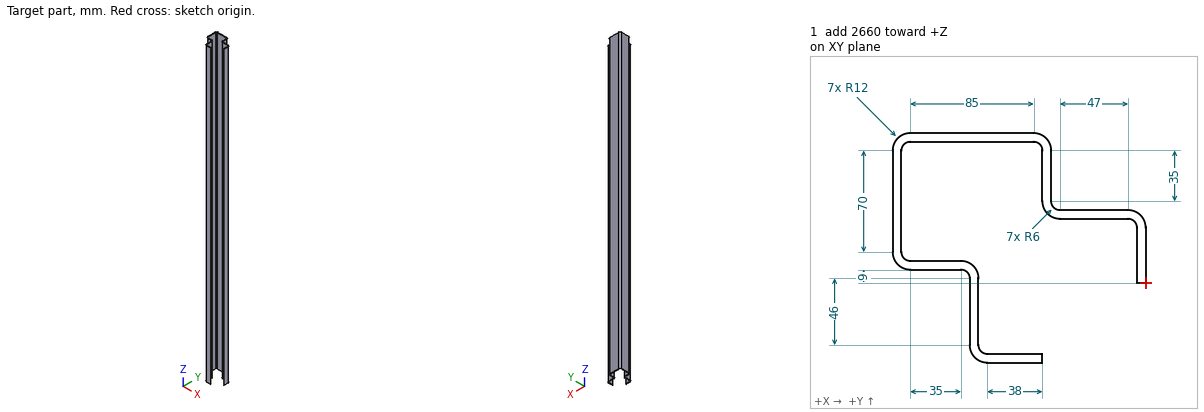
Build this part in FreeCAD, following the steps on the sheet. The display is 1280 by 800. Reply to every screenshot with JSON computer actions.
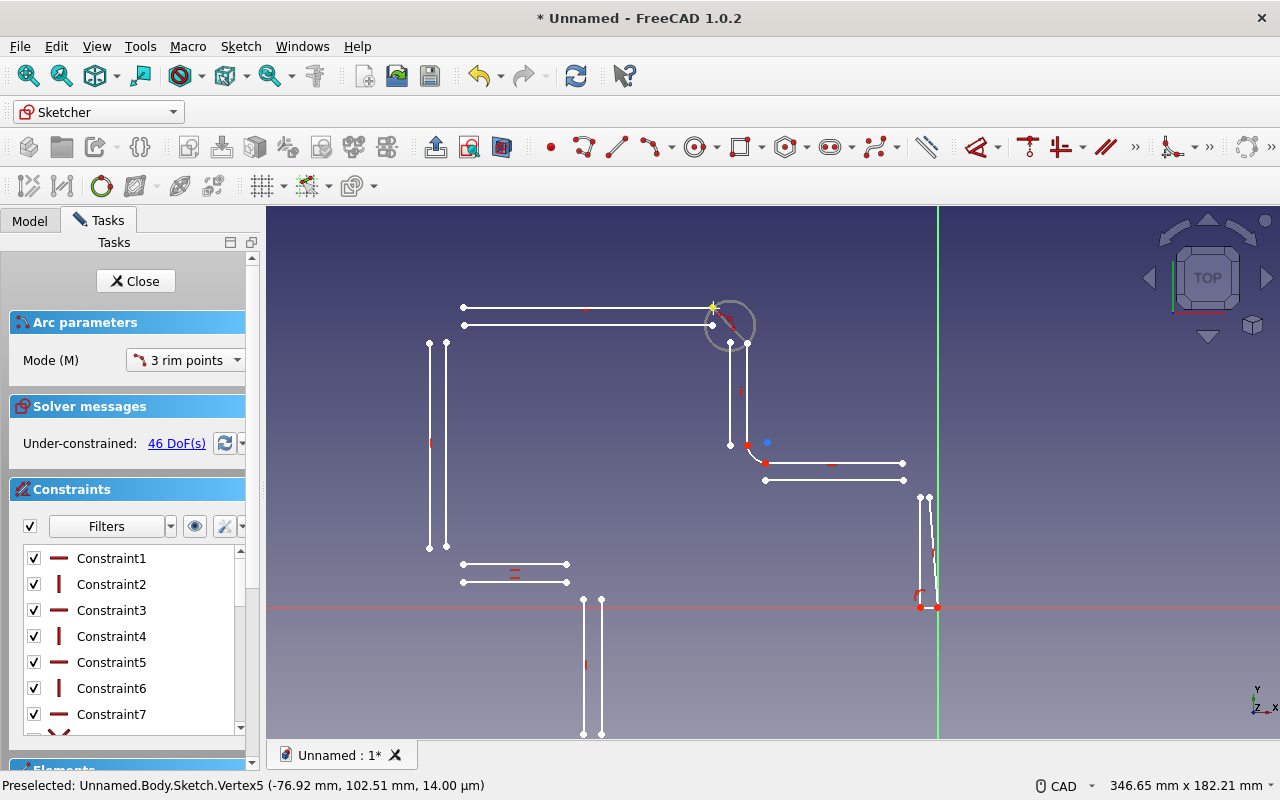
{"action": "scroll", "coordinate": [738, 317], "scroll_direction": "up", "scroll_amount": 3}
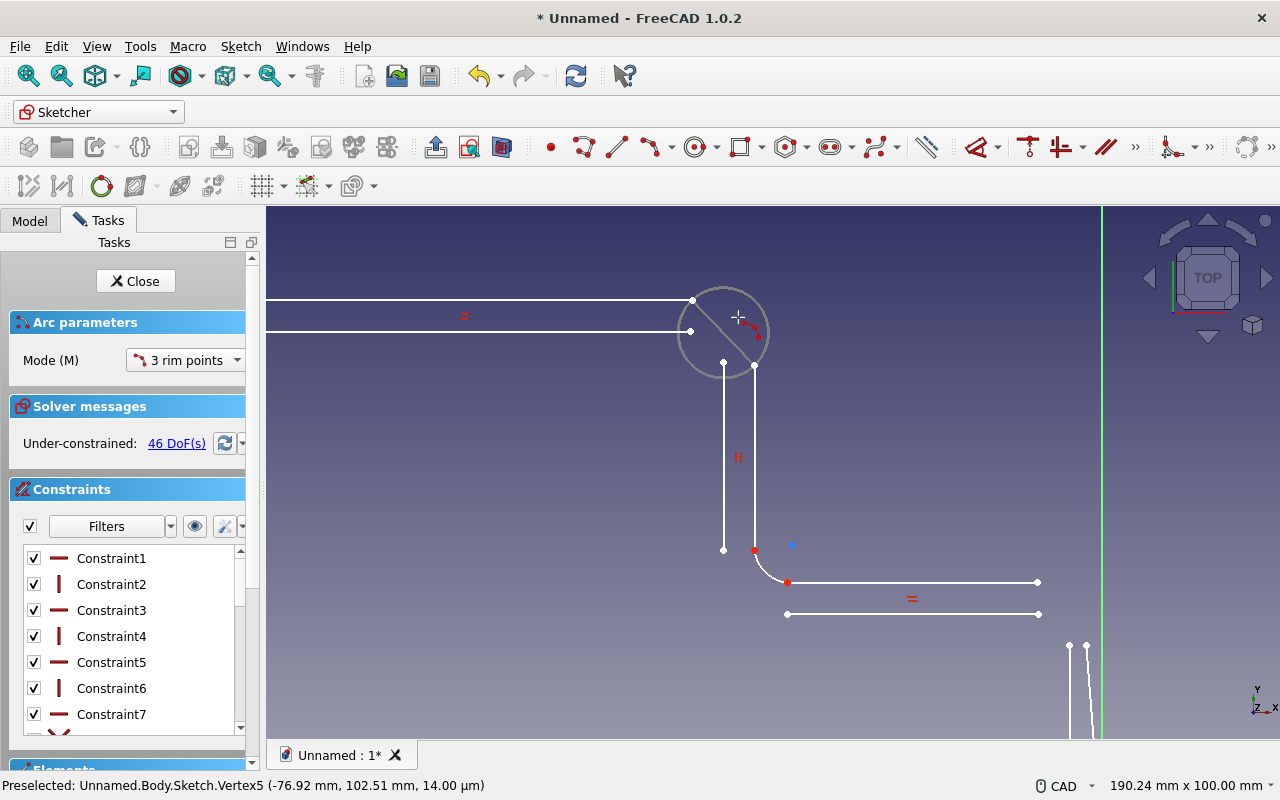
{"action": "left_click", "coordinate": [737, 316]}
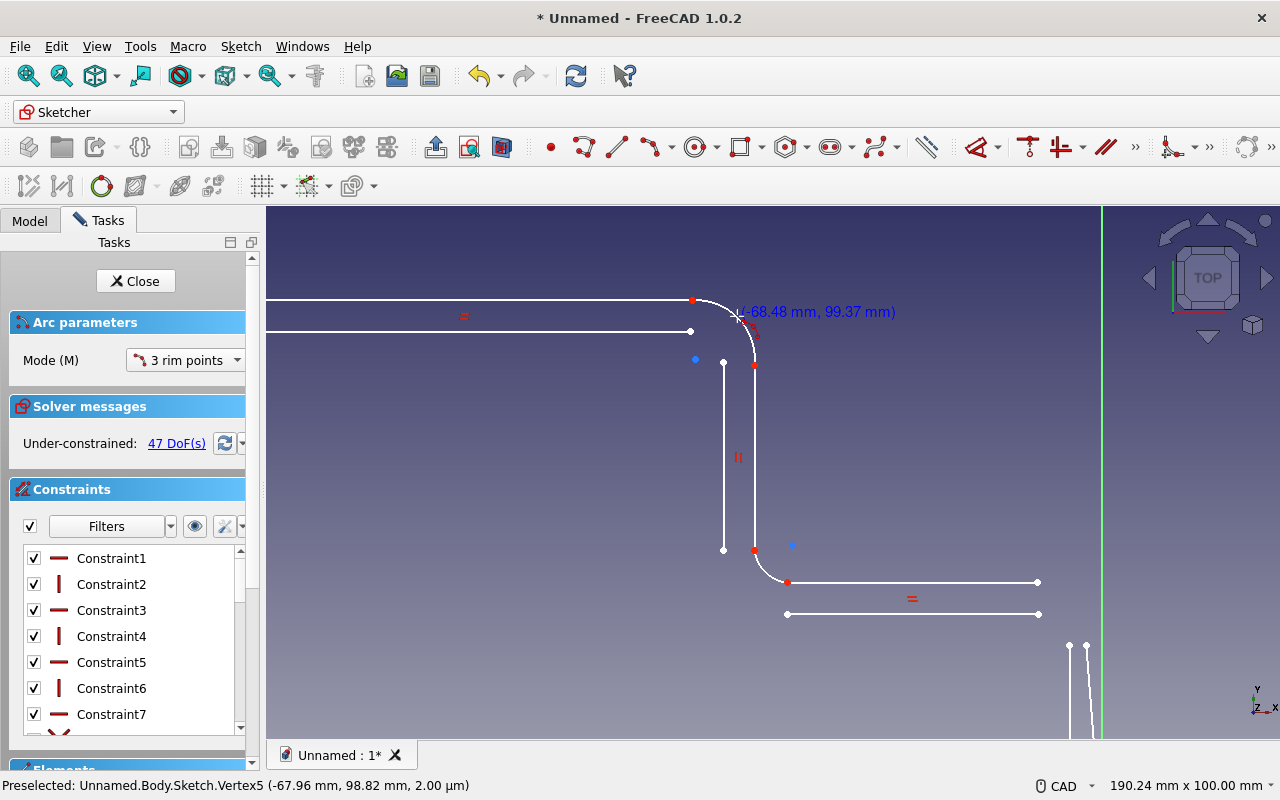
{"action": "scroll", "coordinate": [743, 329], "scroll_direction": "down", "scroll_amount": 5}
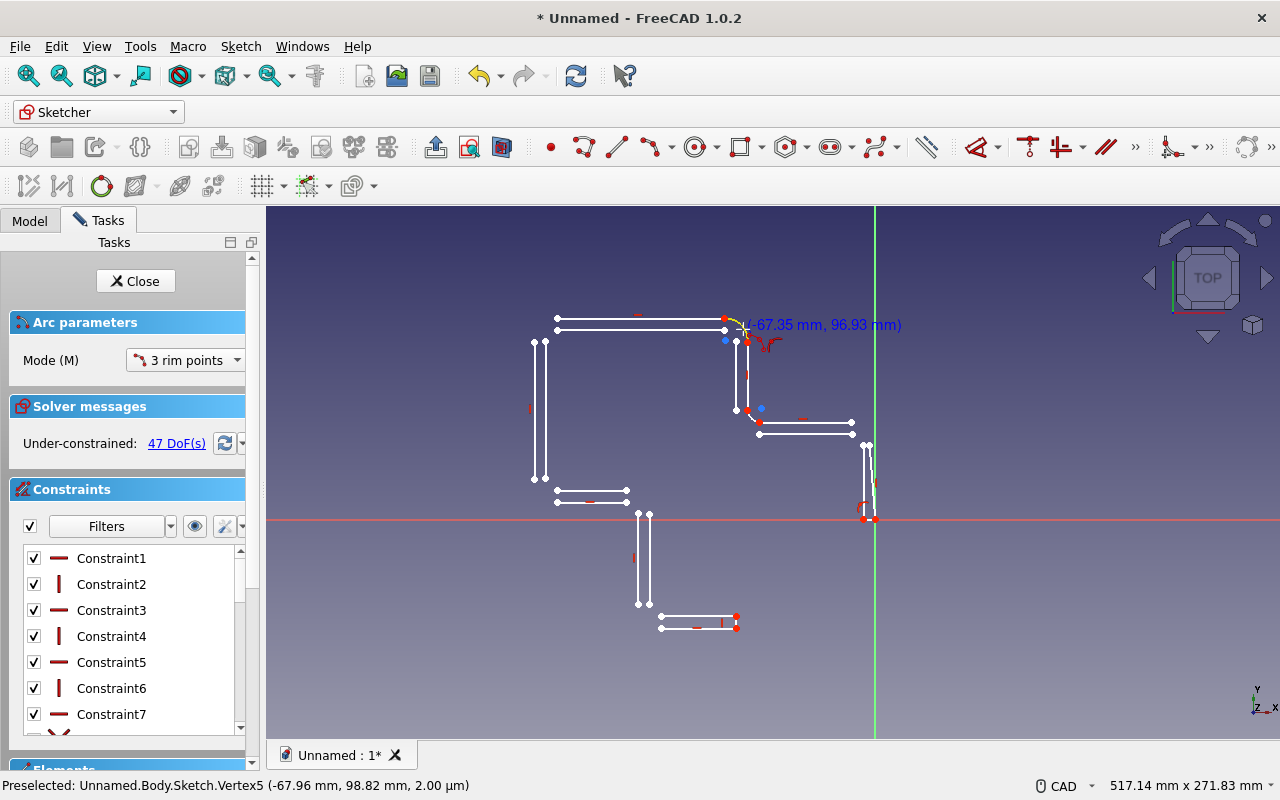
{"action": "scroll", "coordinate": [558, 318], "scroll_direction": "up", "scroll_amount": 2}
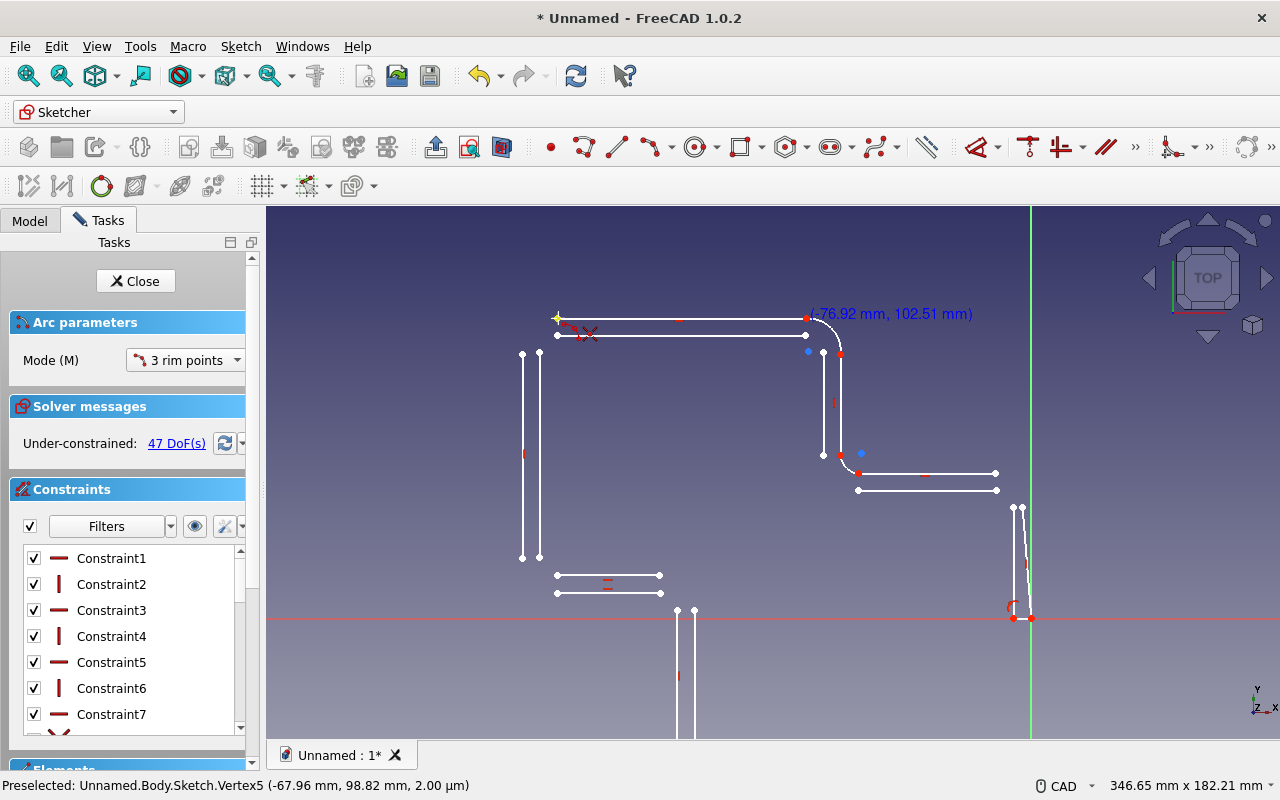
{"action": "left_click", "coordinate": [557, 319]}
{"action": "left_click", "coordinate": [523, 355]}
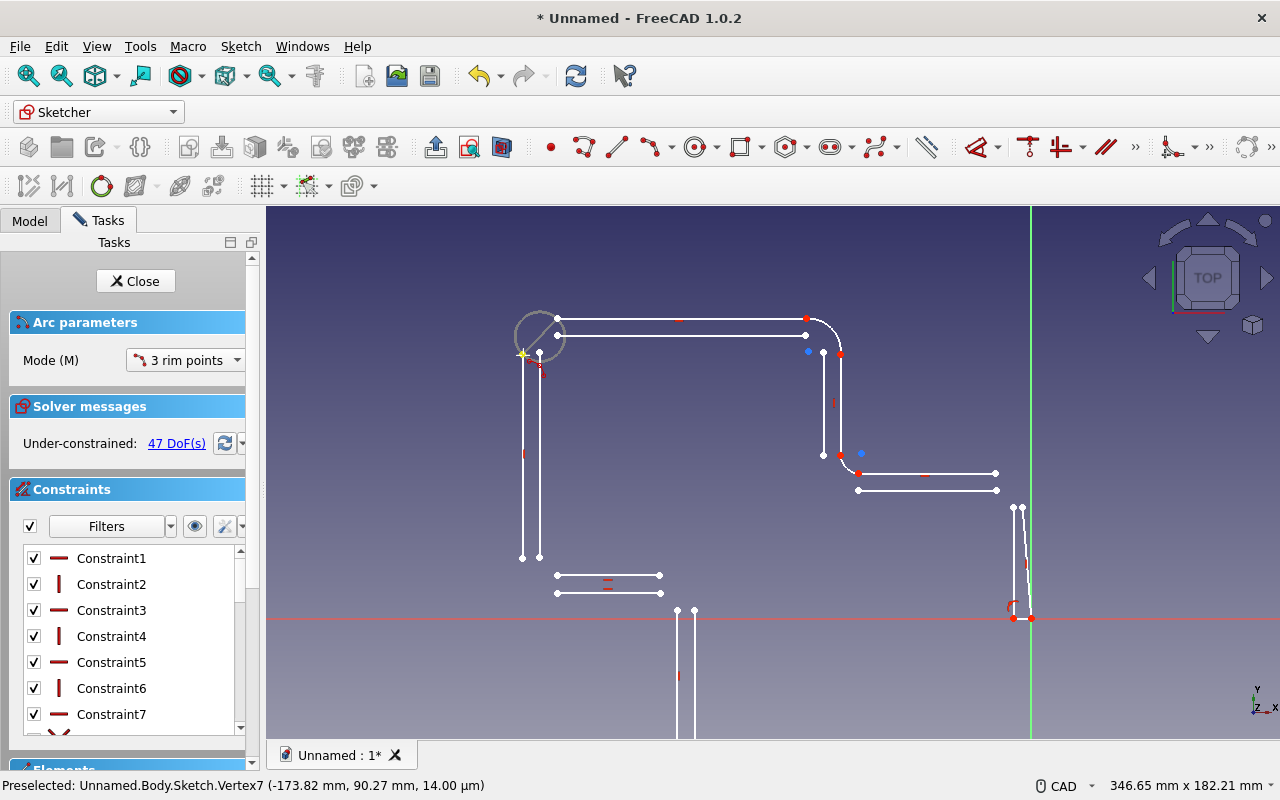
{"action": "scroll", "coordinate": [533, 328], "scroll_direction": "up", "scroll_amount": 3}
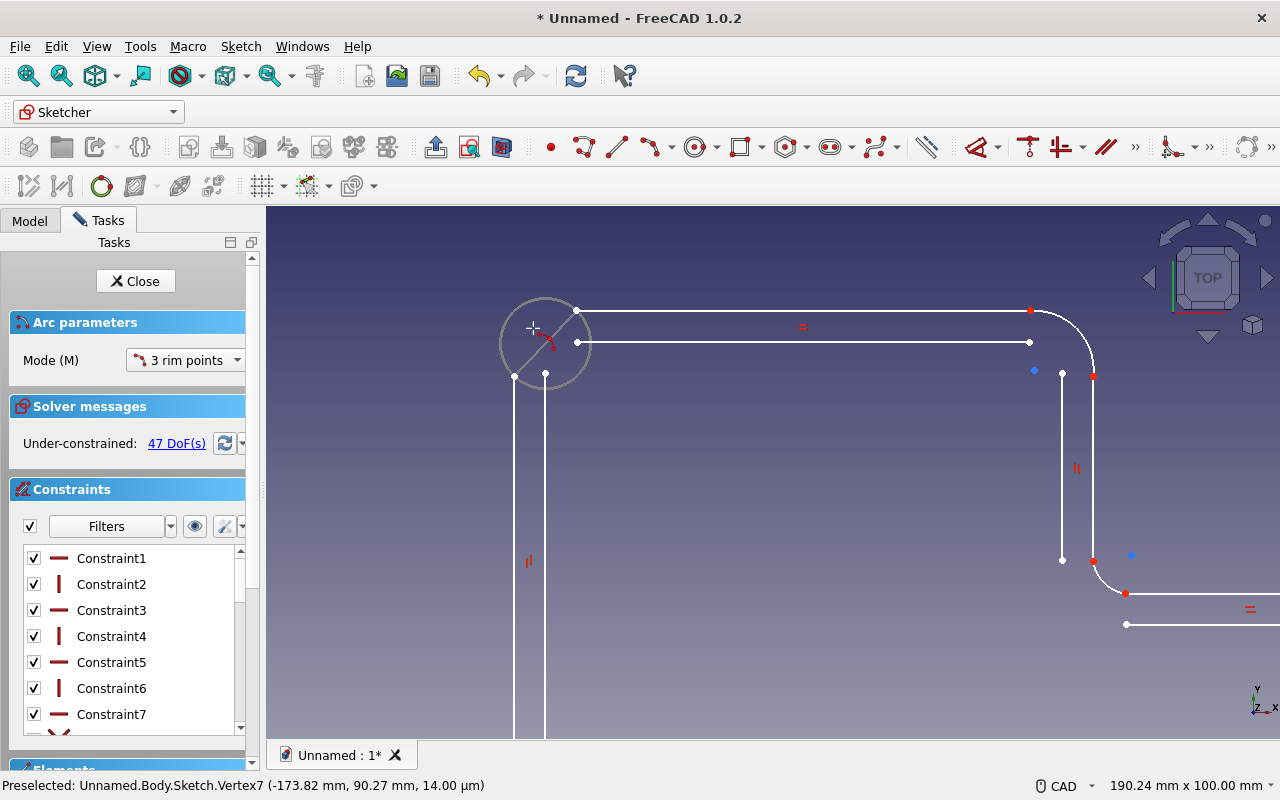
{"action": "left_click", "coordinate": [532, 327]}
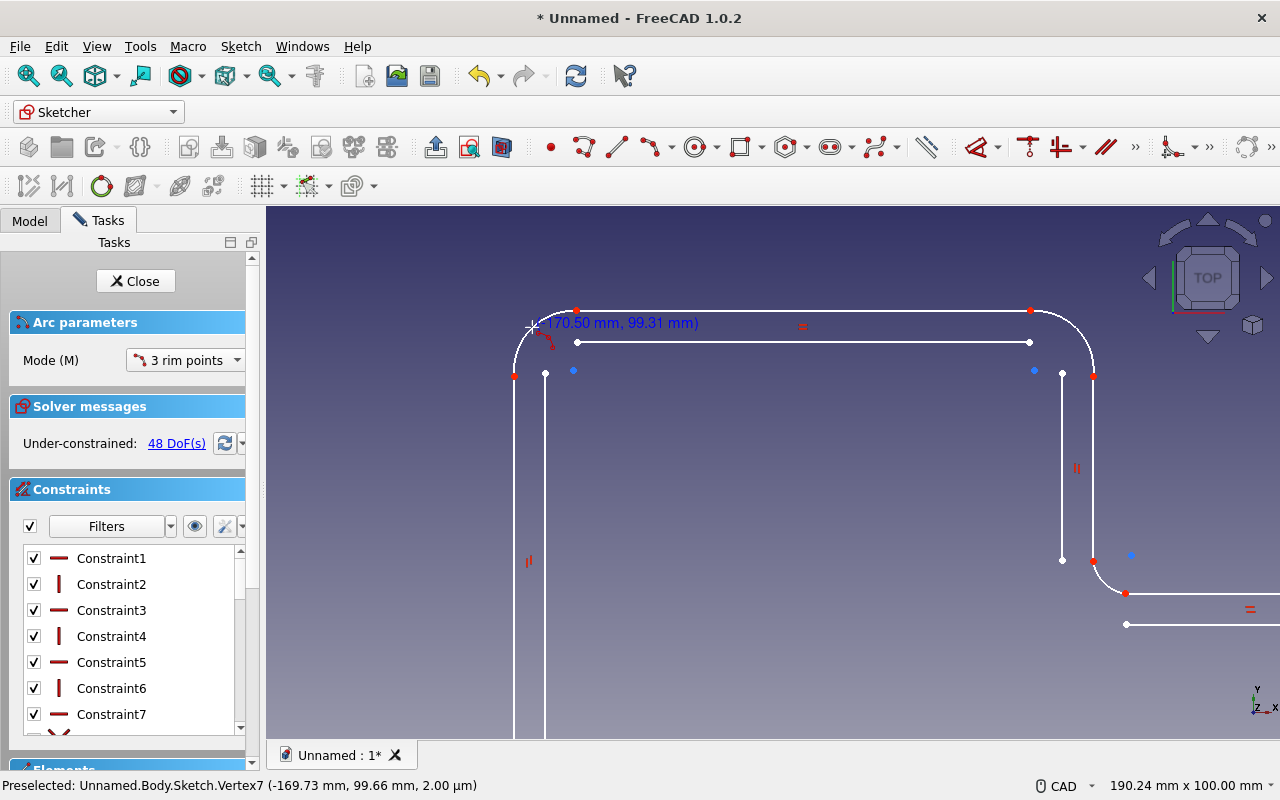
{"action": "scroll", "coordinate": [546, 323], "scroll_direction": "down", "scroll_amount": 5}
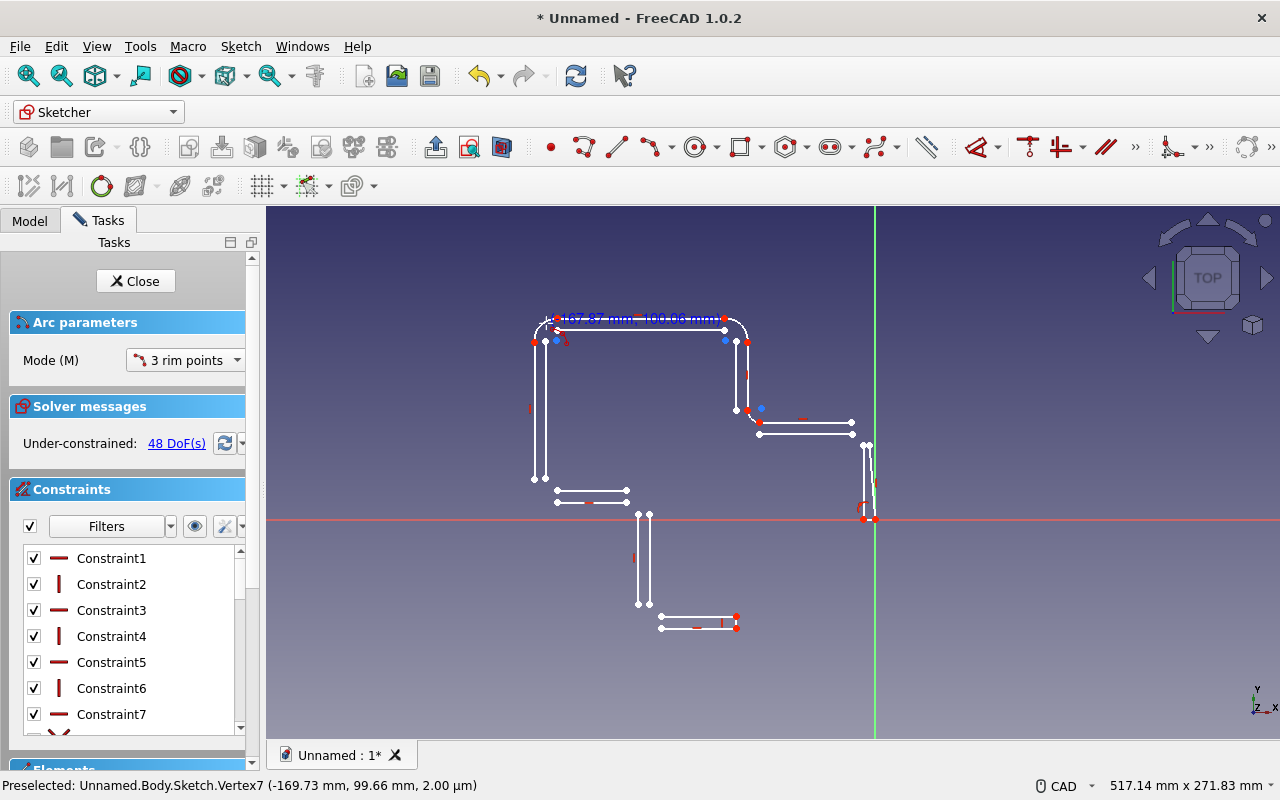
{"action": "scroll", "coordinate": [534, 479], "scroll_direction": "up", "scroll_amount": 2}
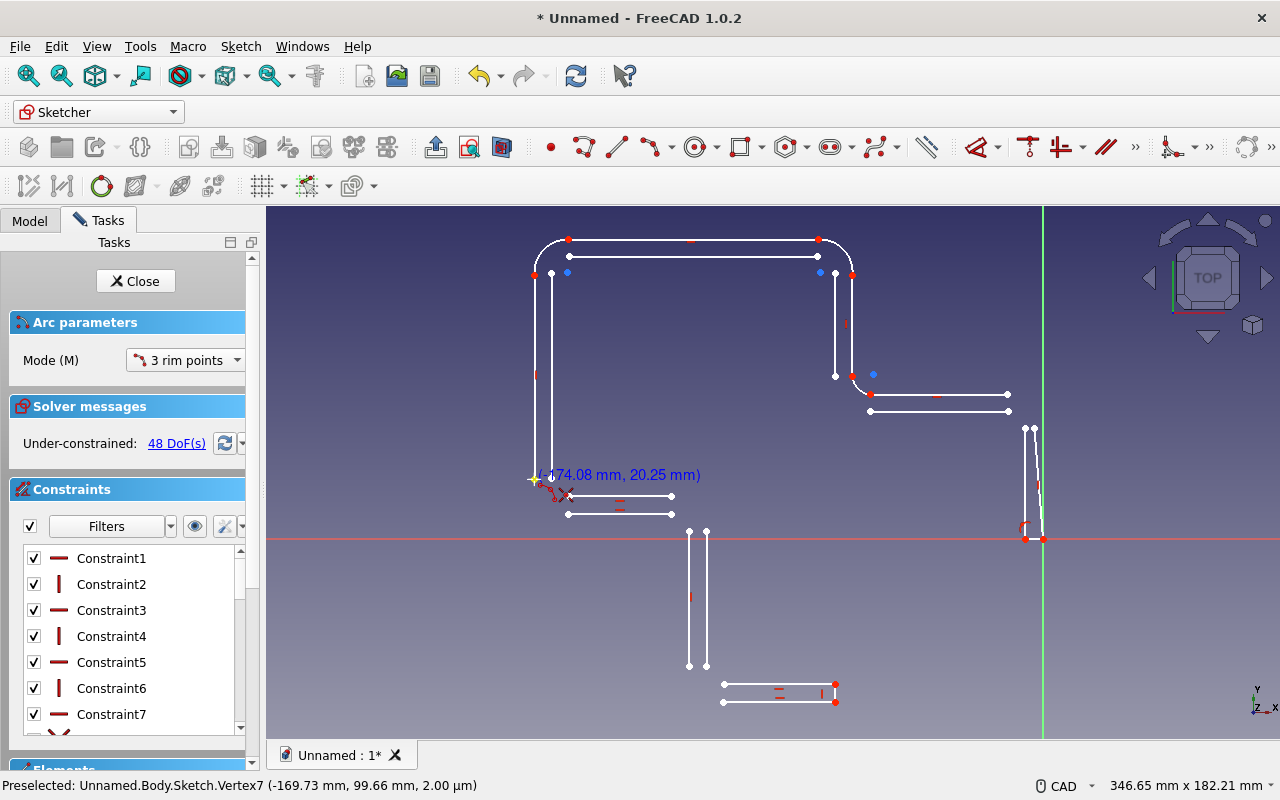
{"action": "left_click", "coordinate": [535, 480]}
{"action": "left_click", "coordinate": [569, 514]}